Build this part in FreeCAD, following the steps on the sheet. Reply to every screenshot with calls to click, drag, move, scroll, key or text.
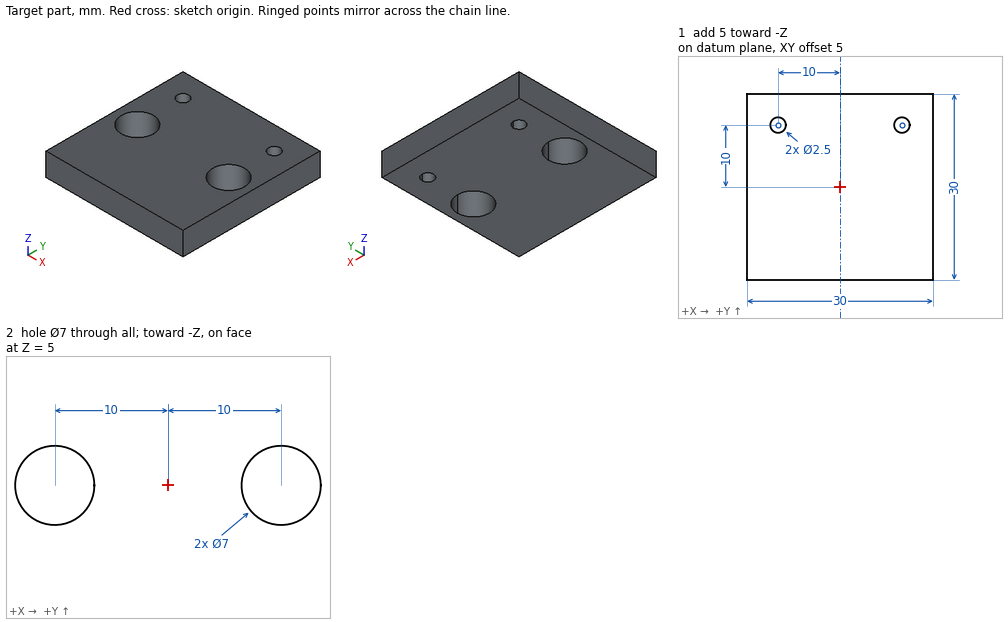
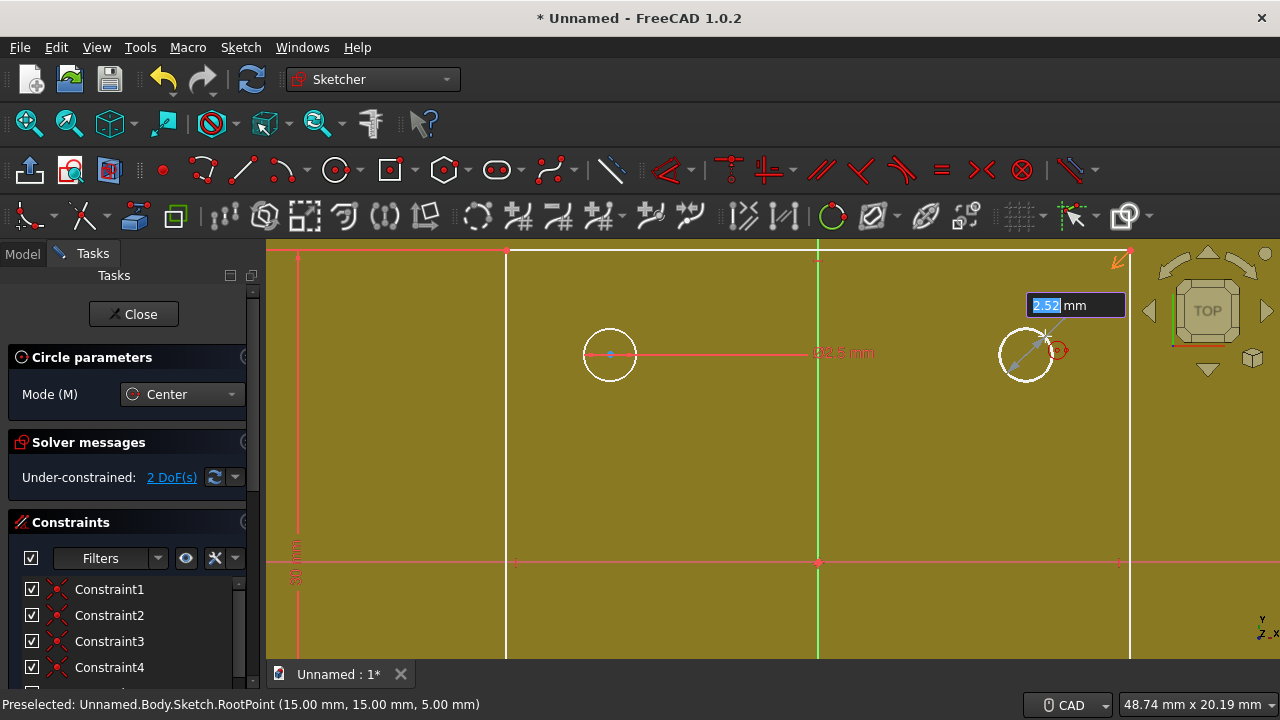
text(2.5)
key(Return)
key(Escape)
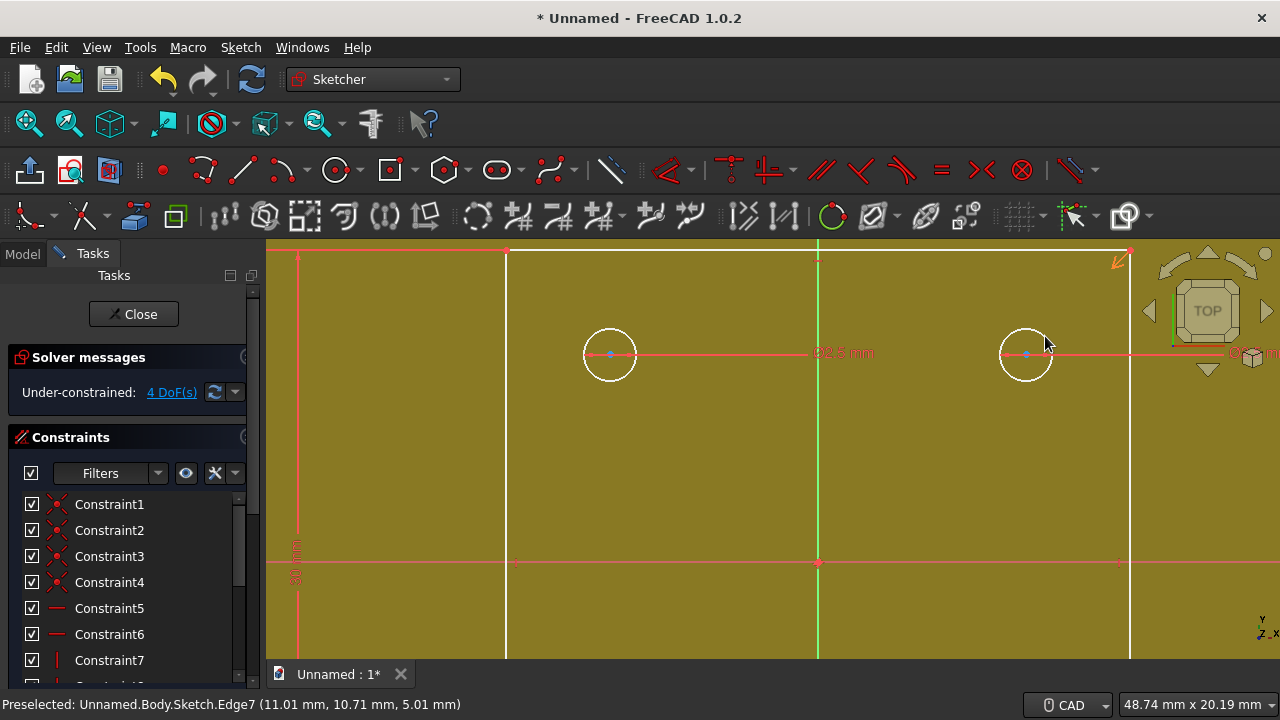
click(610, 355)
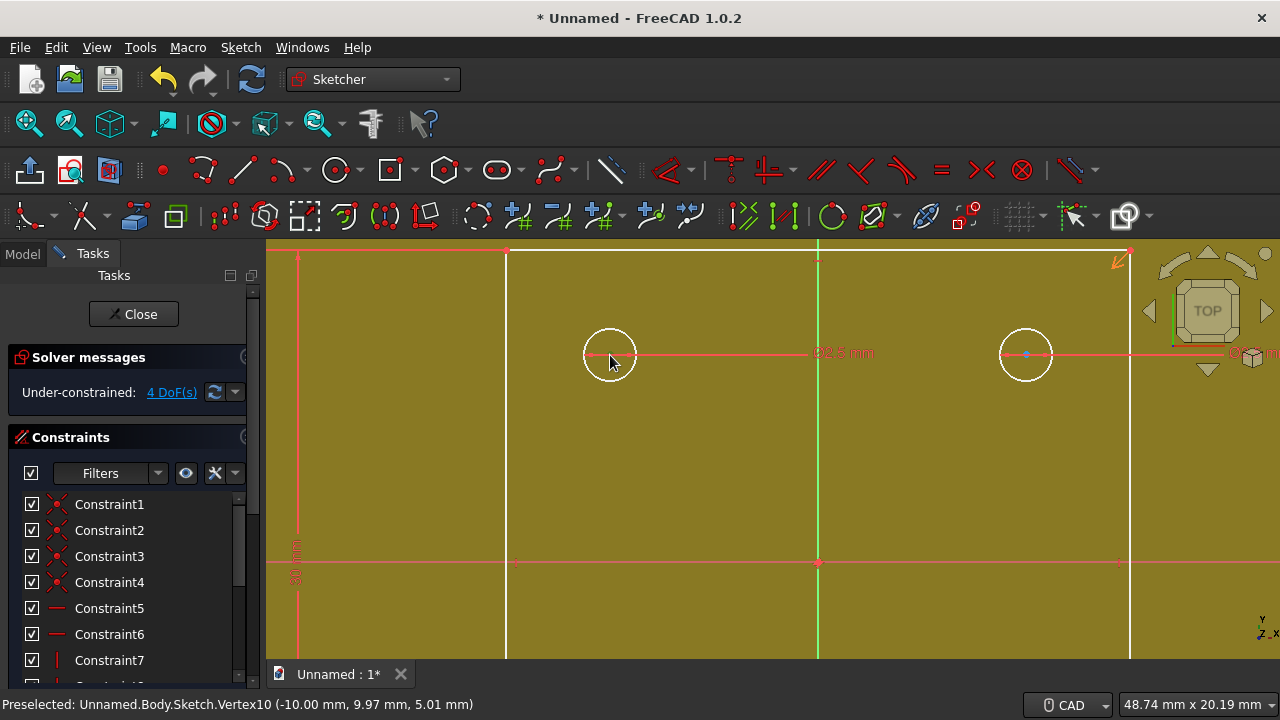
click(1026, 355)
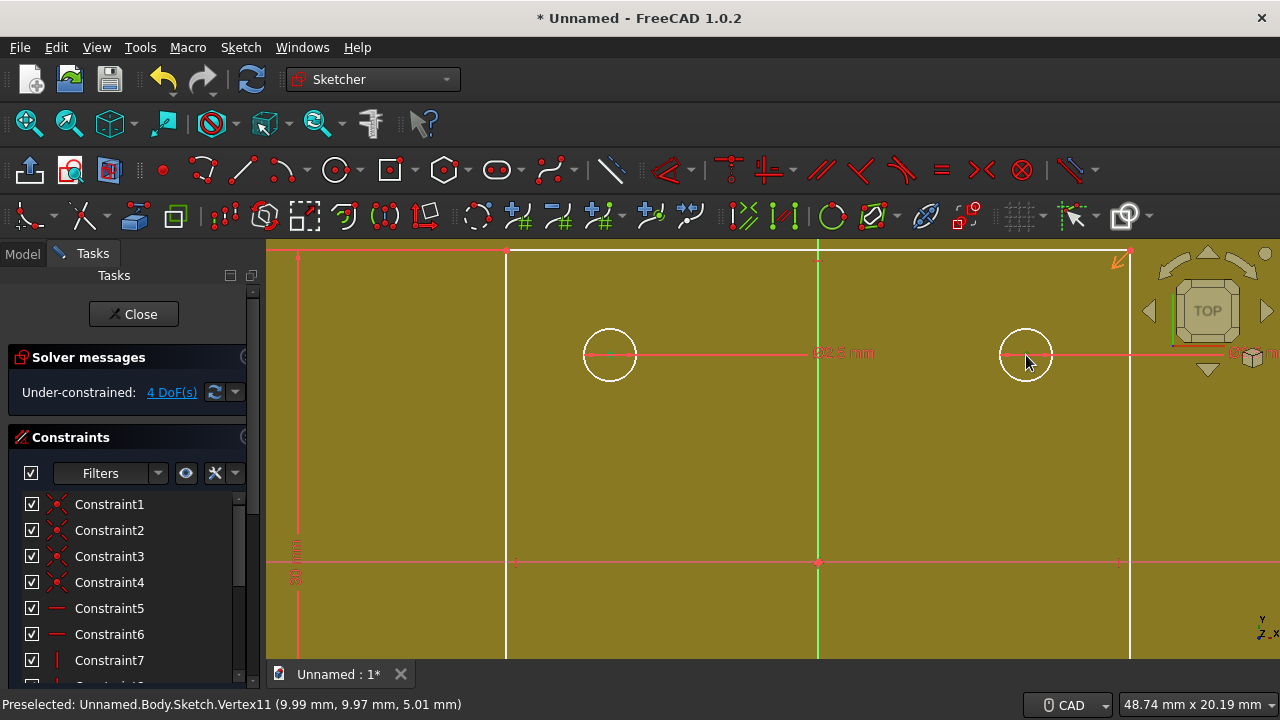
click(818, 605)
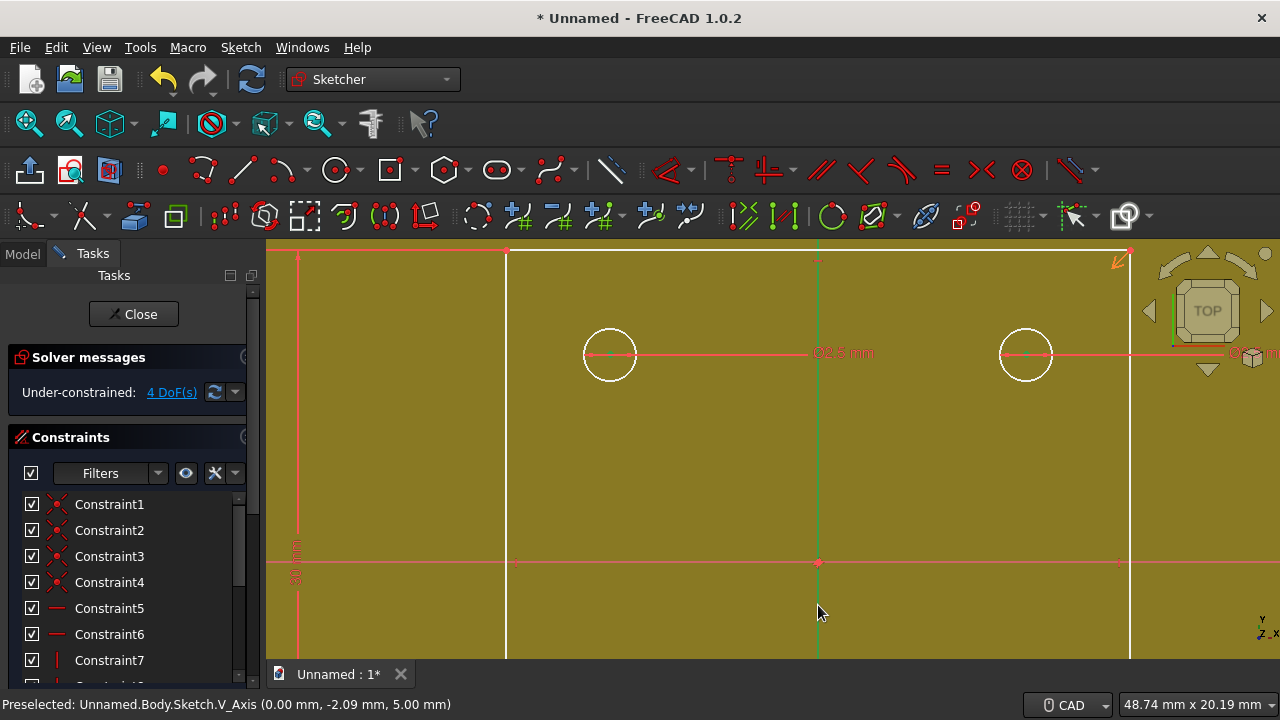
key(s)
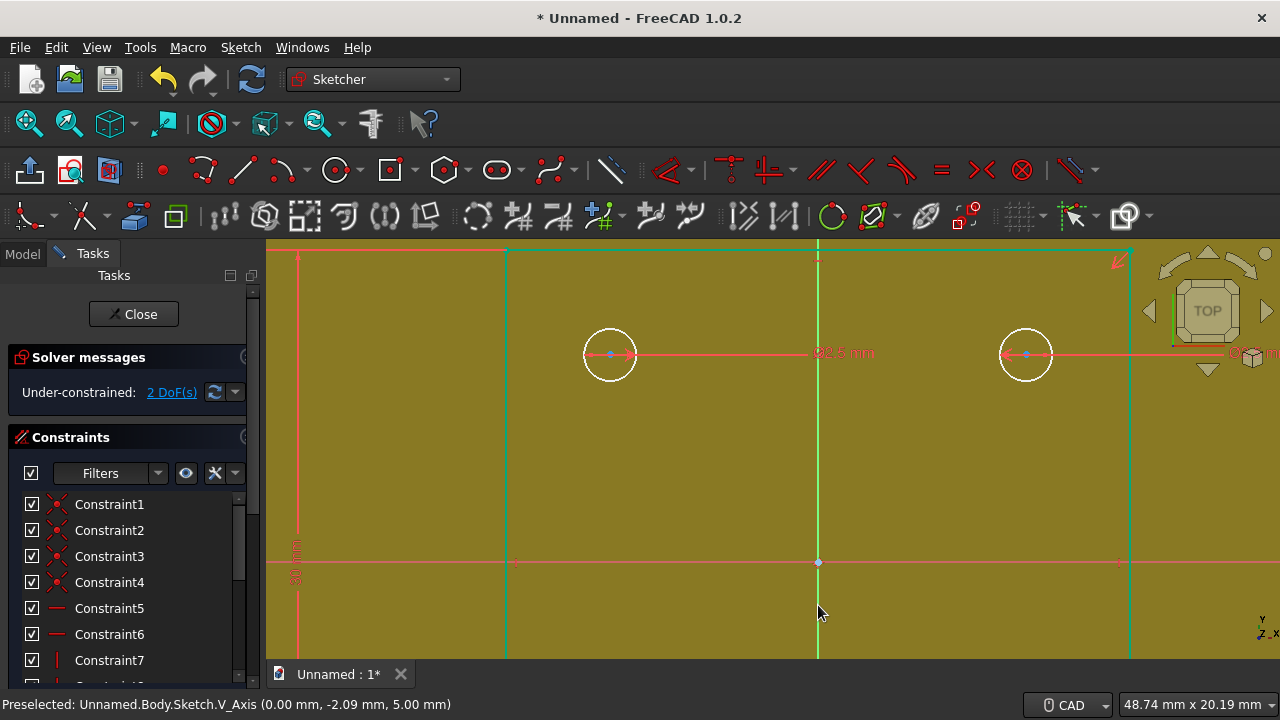
click(666, 170)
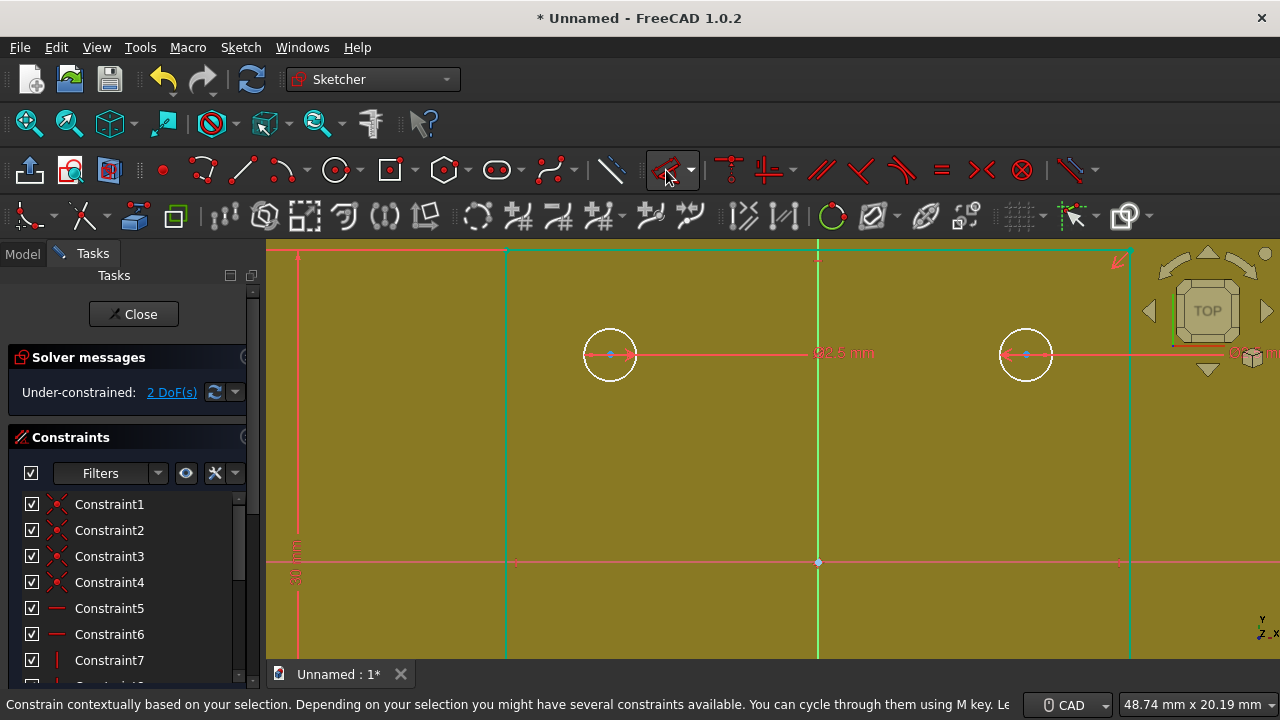
click(610, 355)
click(714, 321)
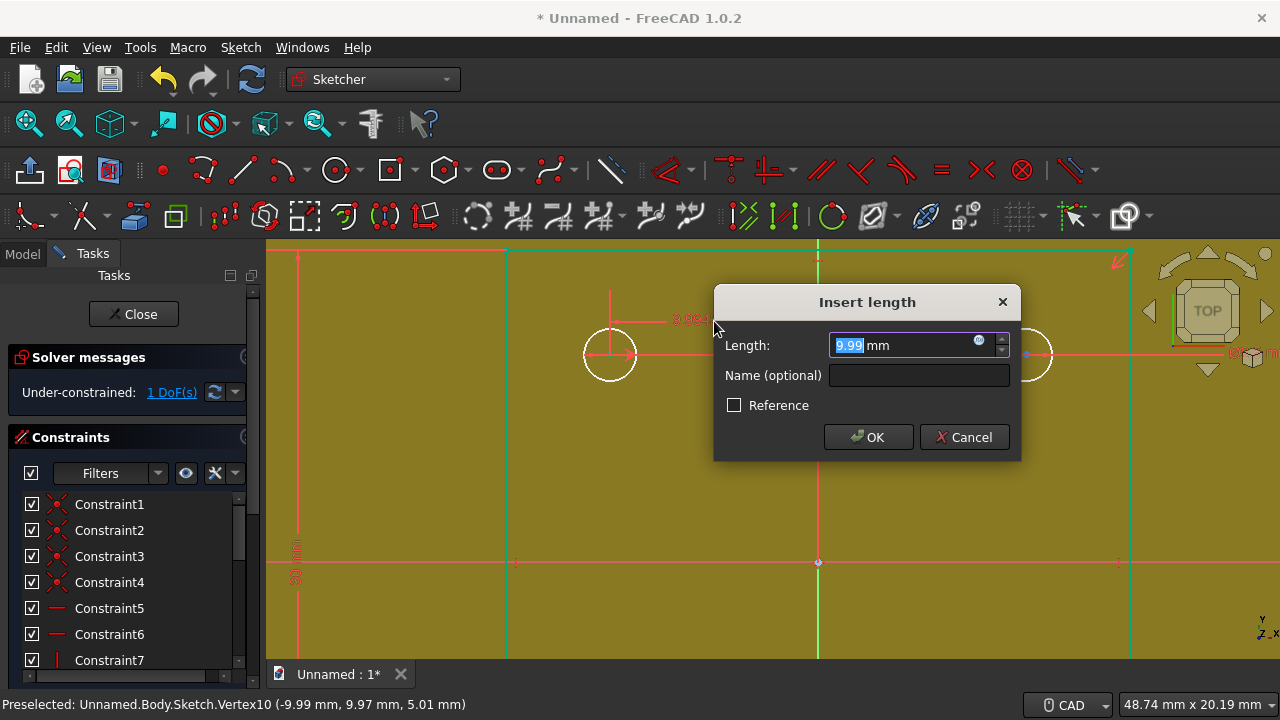
text(10)
key(Return)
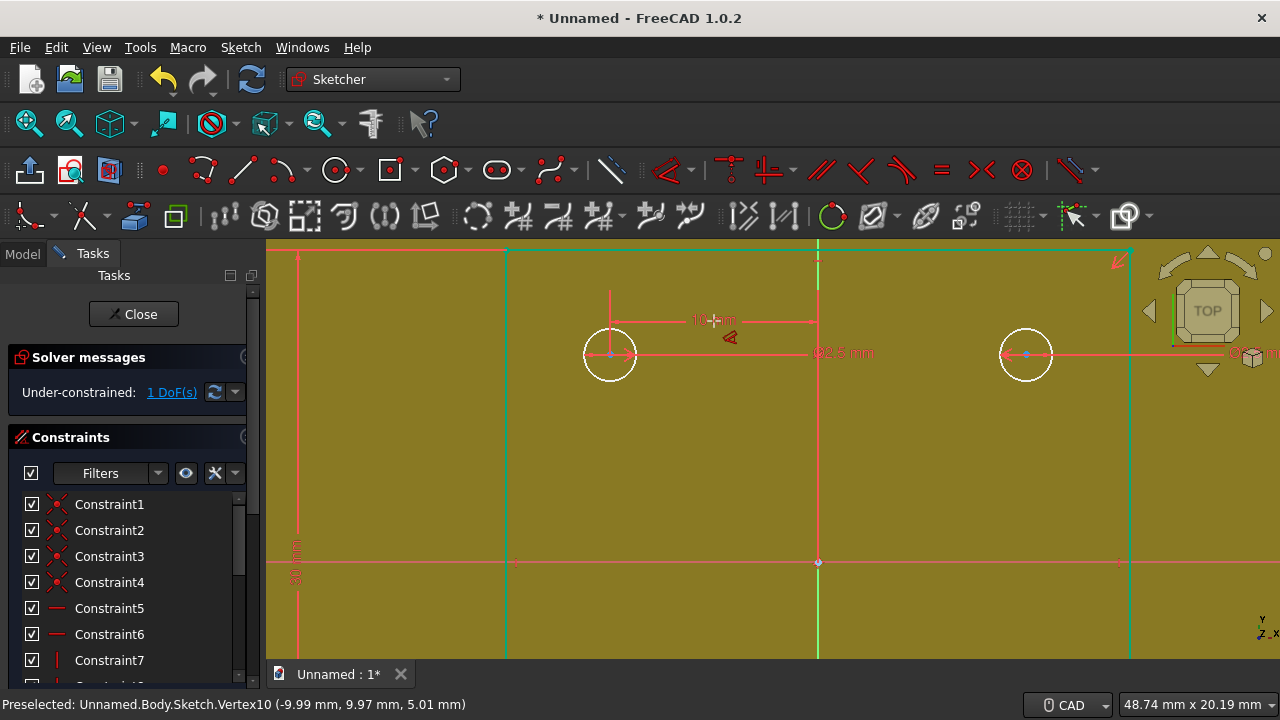
click(610, 355)
click(576, 459)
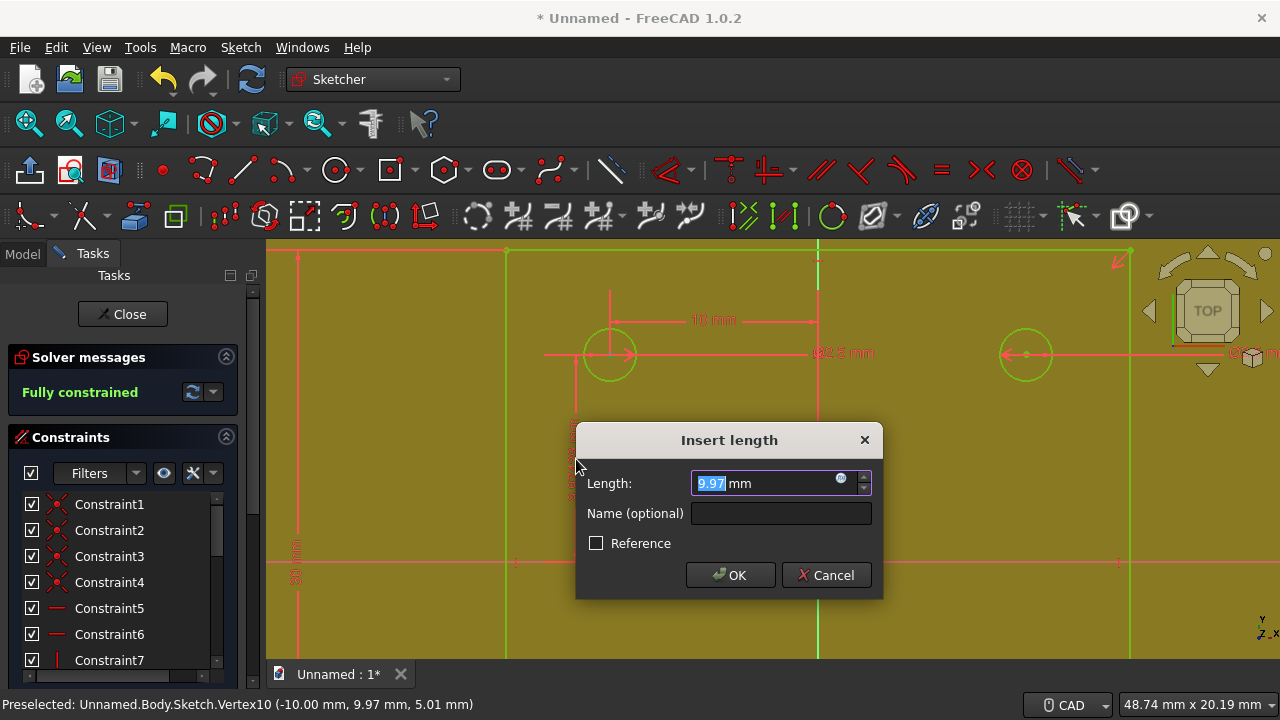
text(10)
key(Return)
key(Escape)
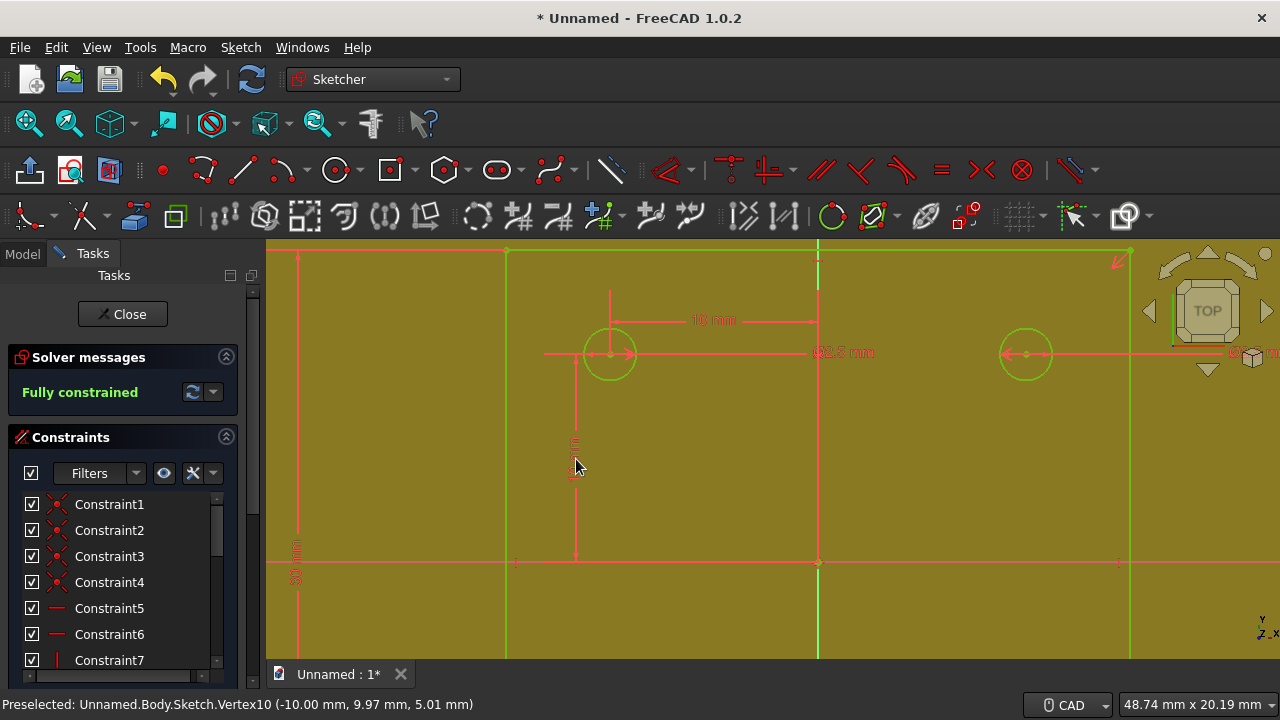
click(123, 314)